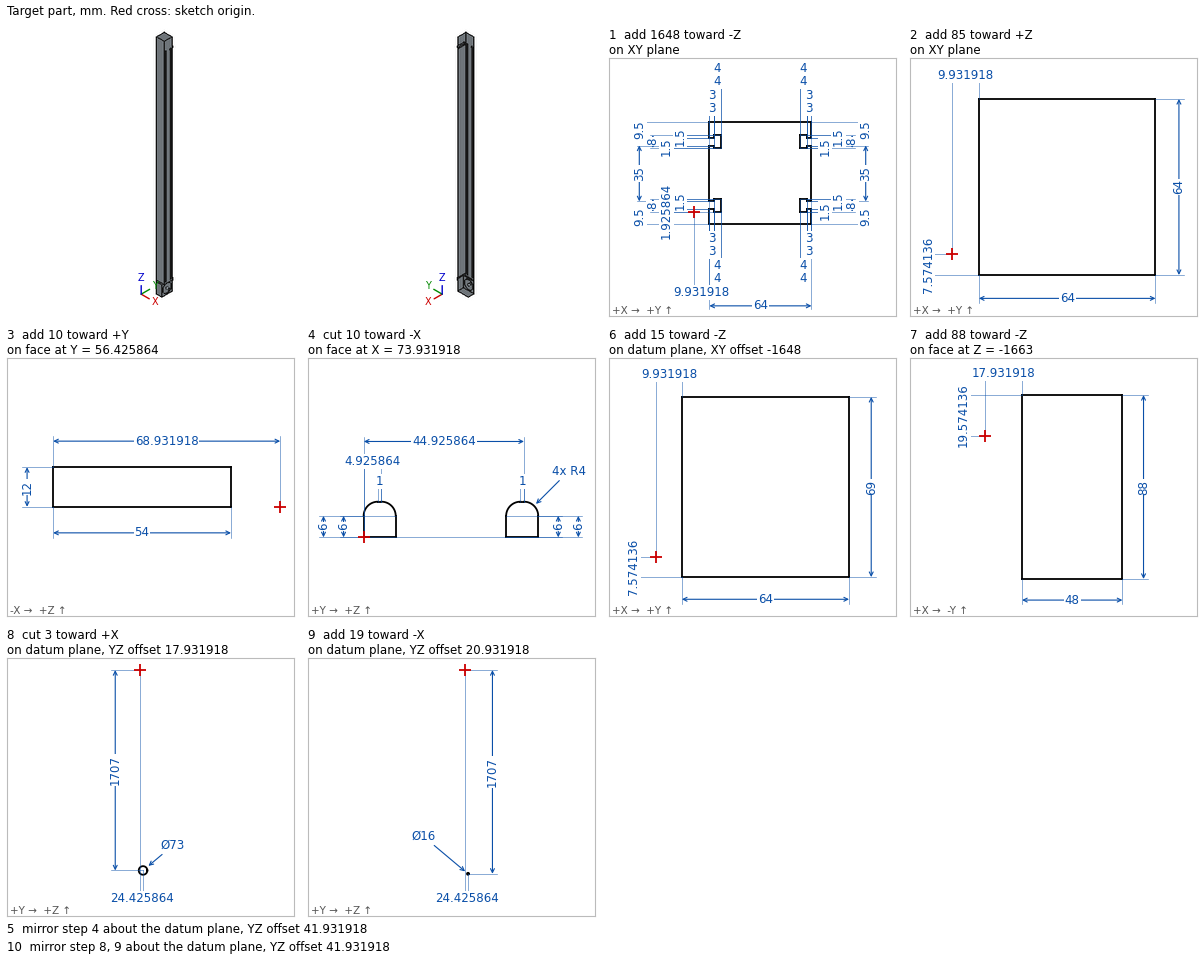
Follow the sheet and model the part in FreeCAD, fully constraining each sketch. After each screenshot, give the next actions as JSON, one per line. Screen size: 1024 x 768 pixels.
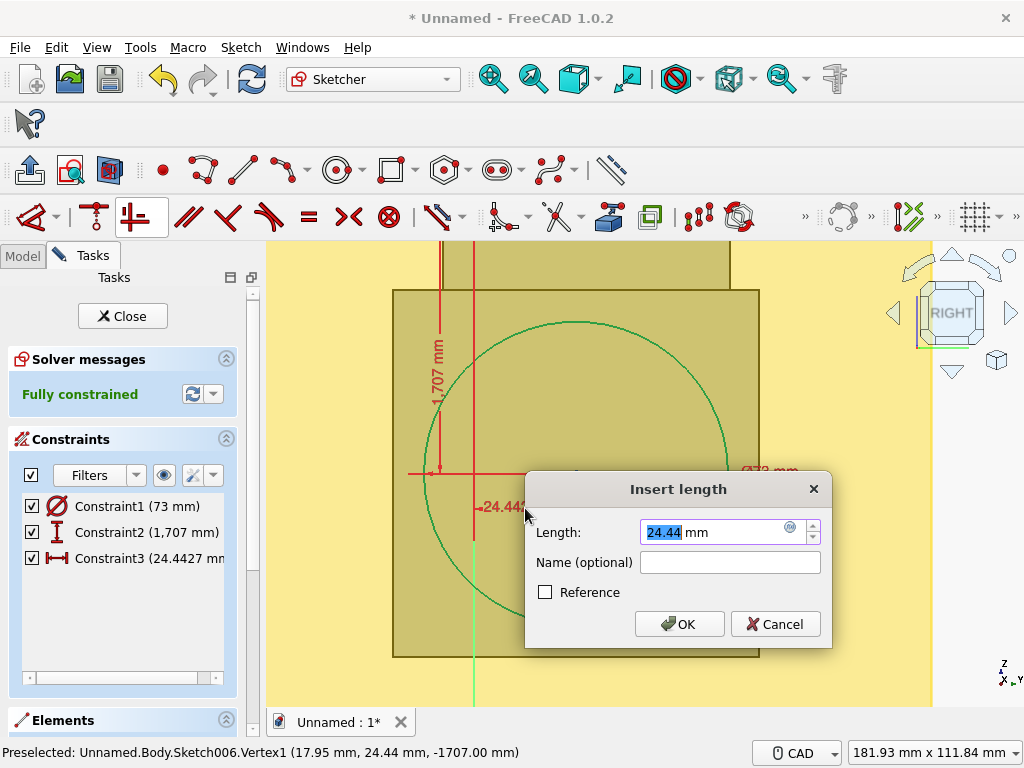
{"action": "type", "text": "24.425864"}
{"action": "key", "text": "Return"}
{"action": "key", "text": "Escape"}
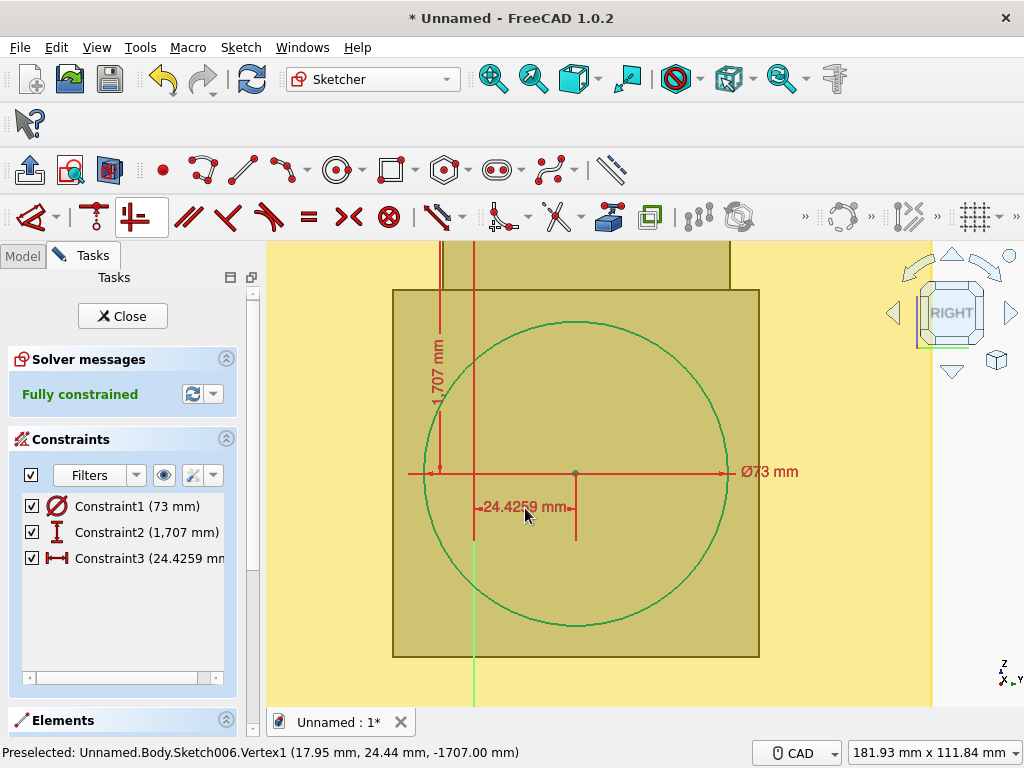
{"action": "left_click", "coordinate": [123, 316]}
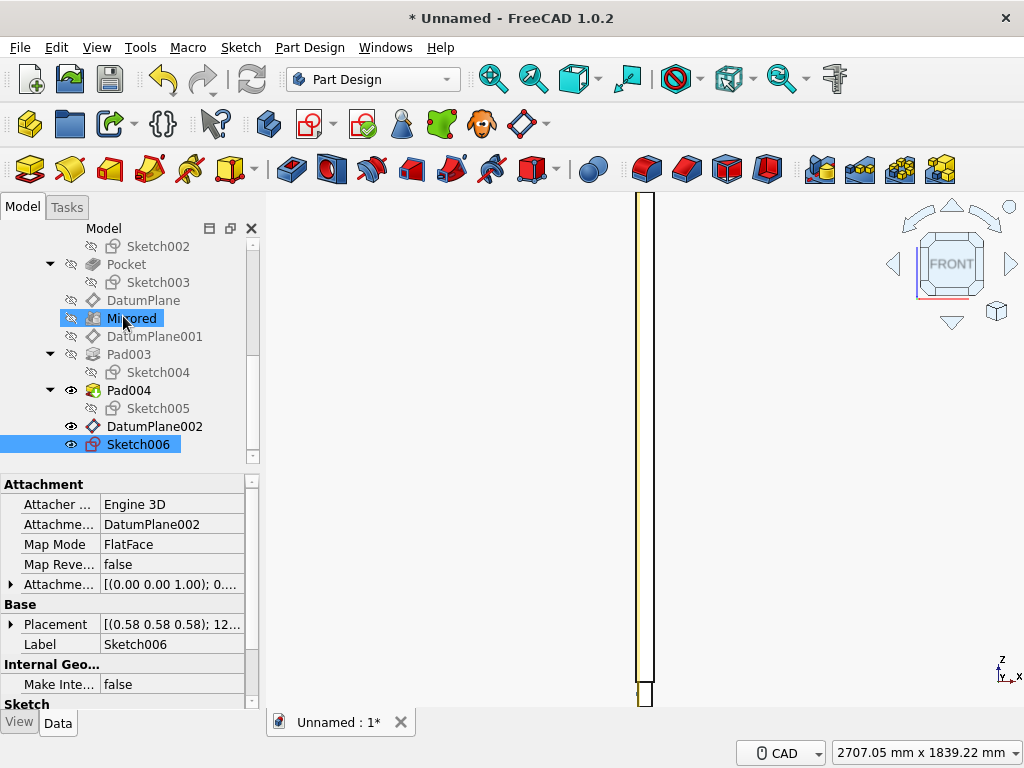
{"action": "left_click", "coordinate": [292, 170]}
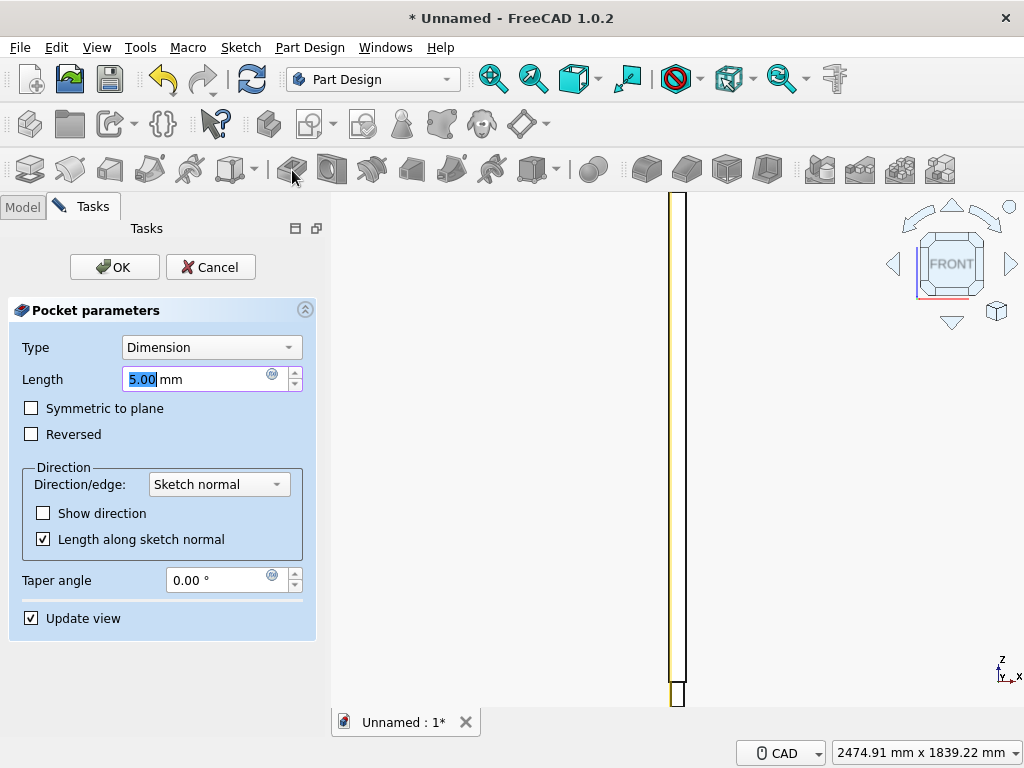
{"action": "type", "text": "3"}
{"action": "key", "text": "Tab"}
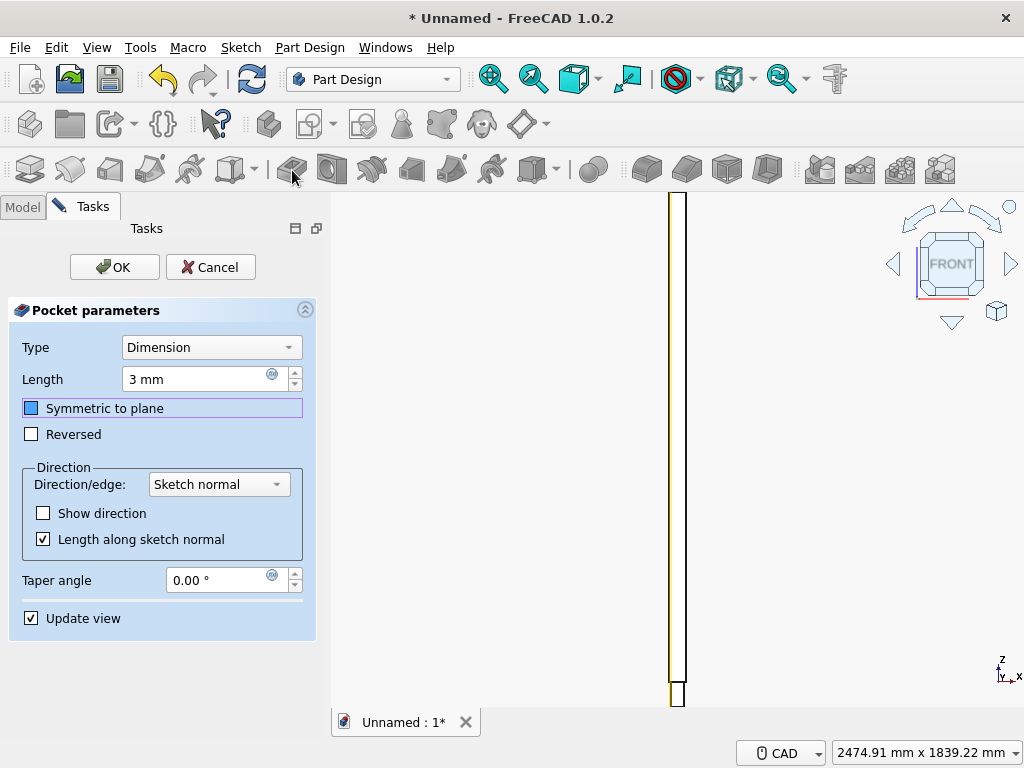
{"action": "left_click", "coordinate": [30, 434]}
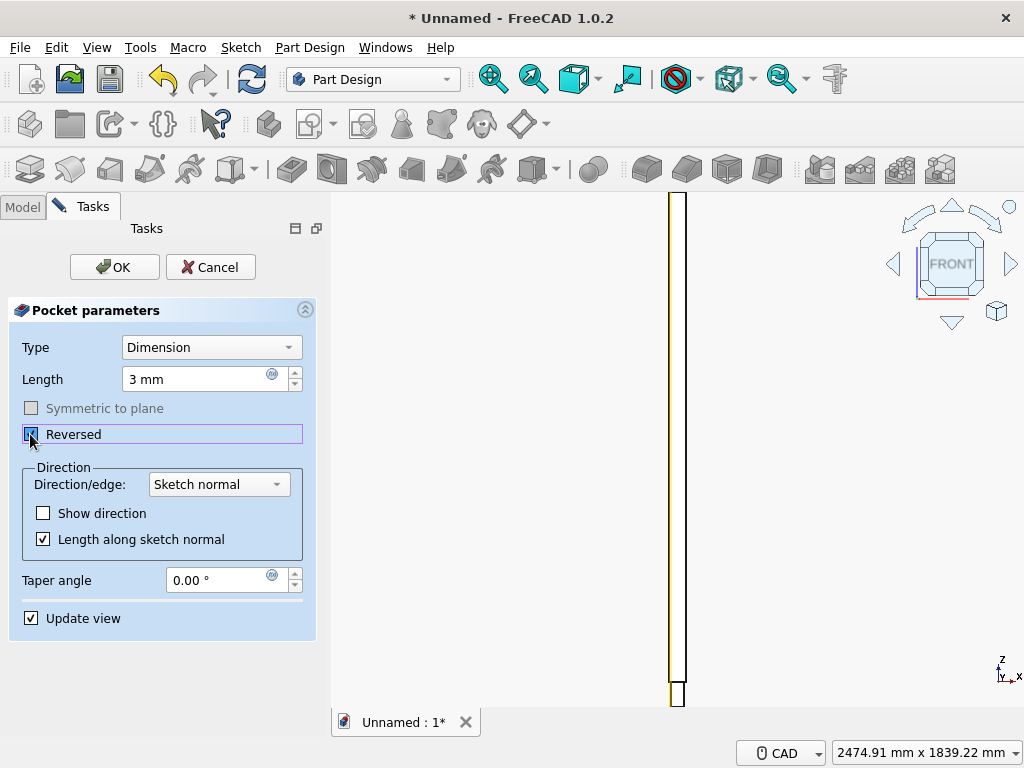
{"action": "left_click", "coordinate": [115, 267]}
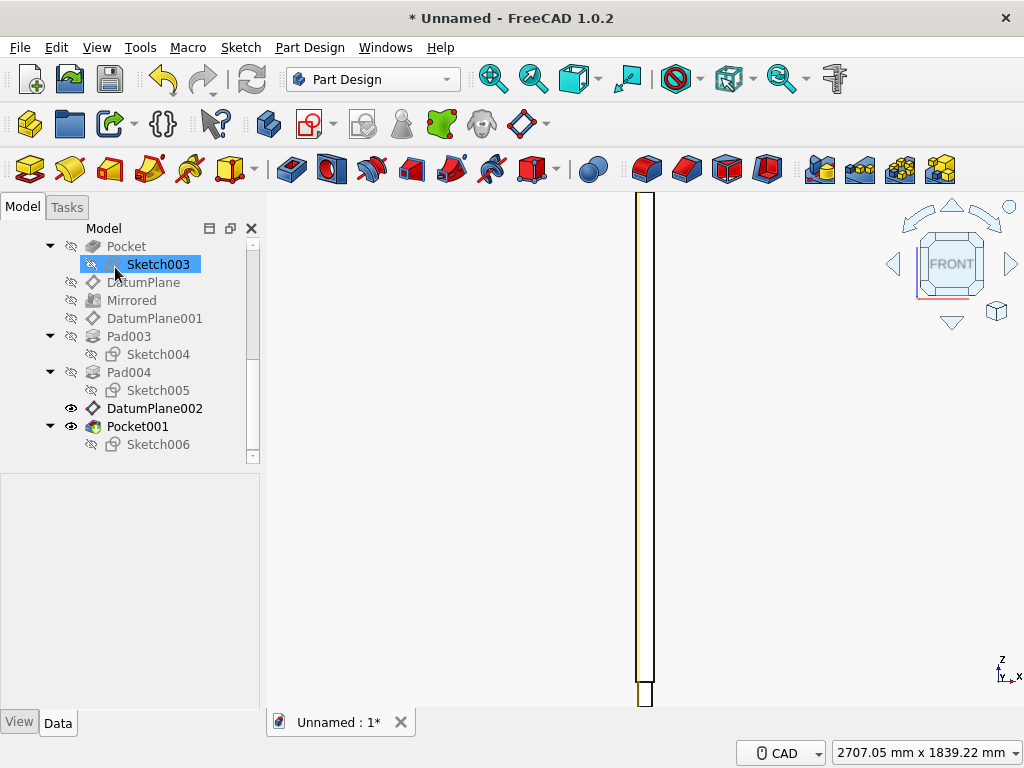
{"action": "left_click", "coordinate": [116, 408]}
{"action": "key", "text": "space"}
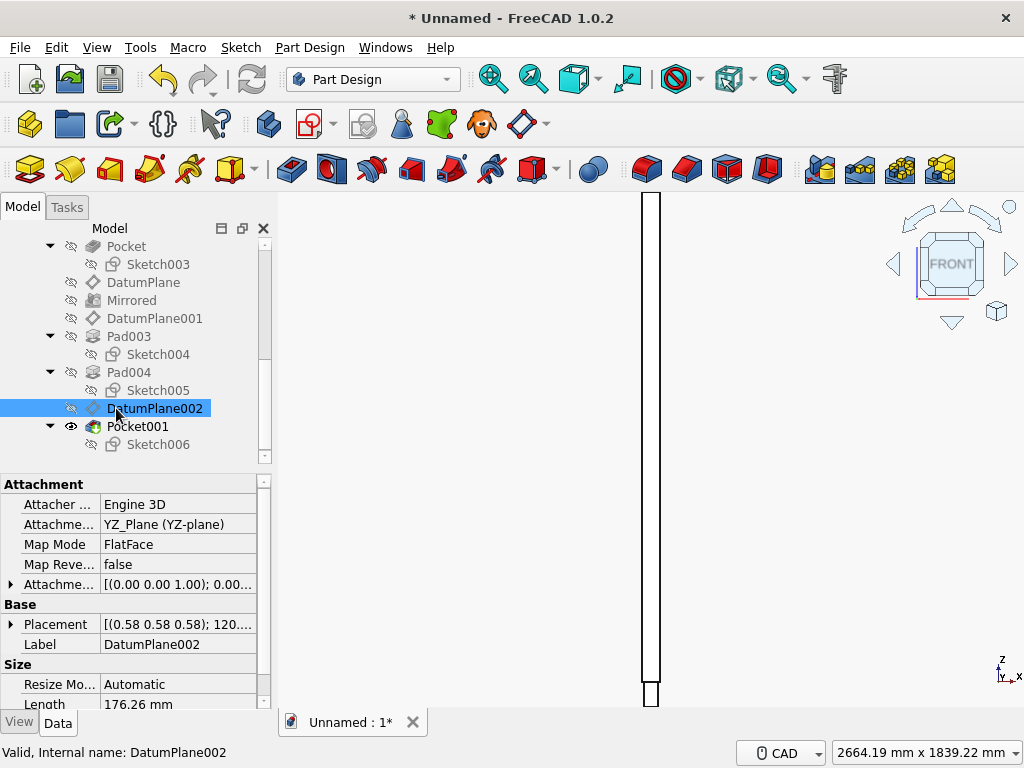
{"action": "left_click", "coordinate": [494, 80]}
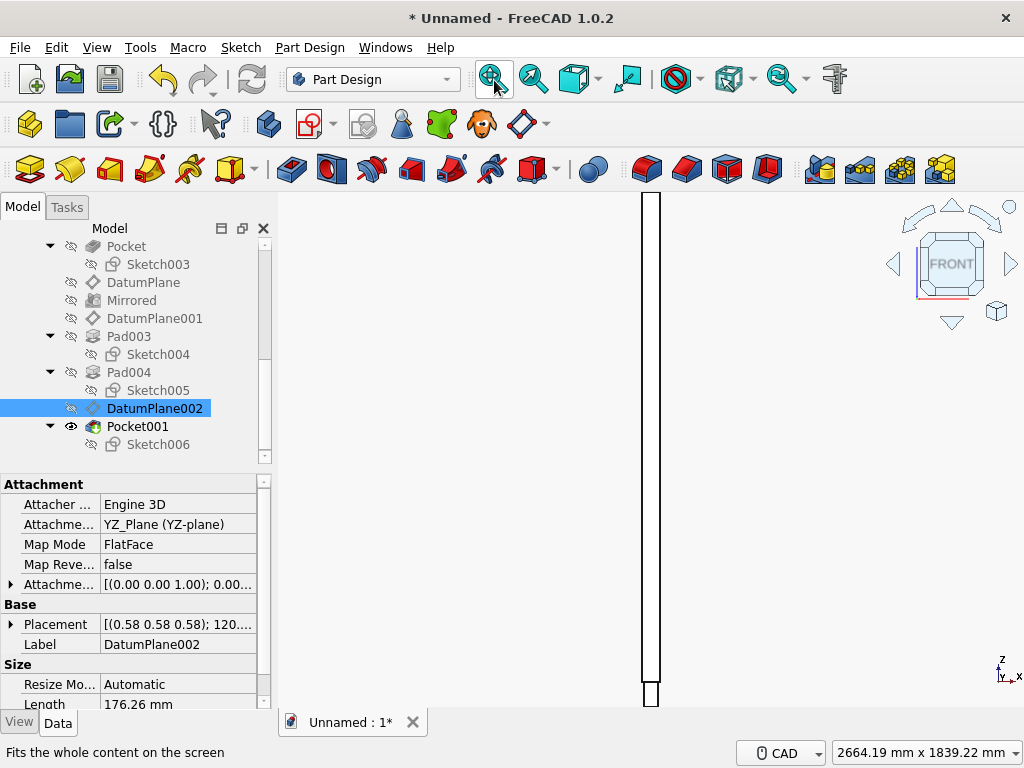
{"action": "key", "text": "6"}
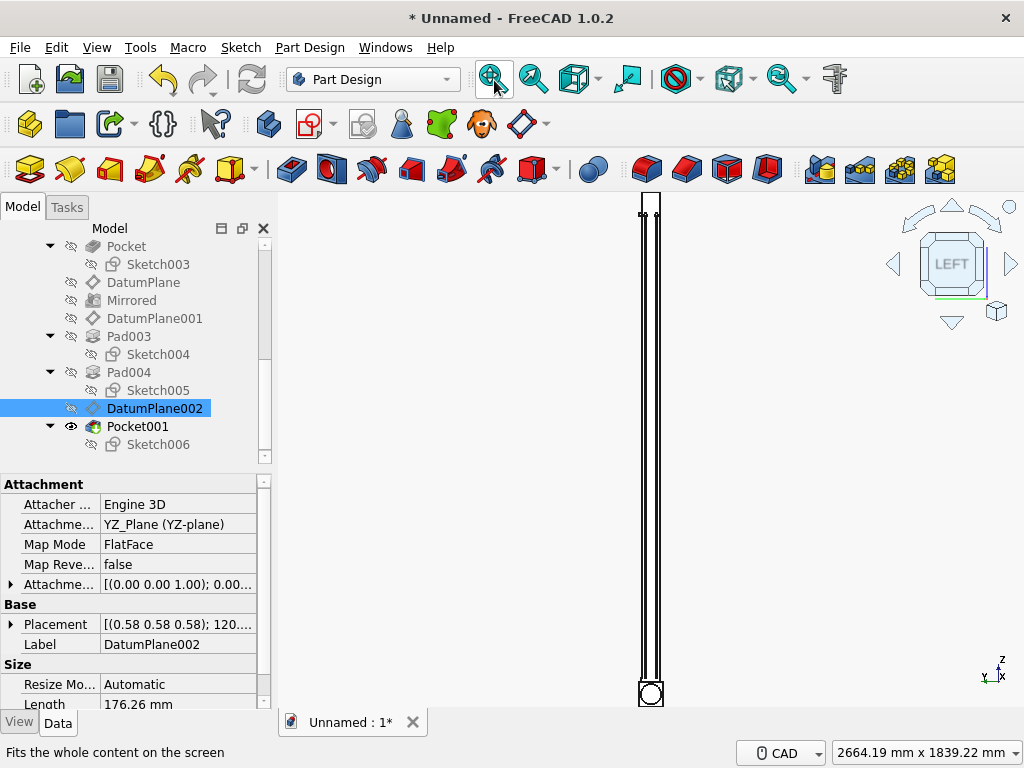
{"action": "left_click", "coordinate": [494, 80]}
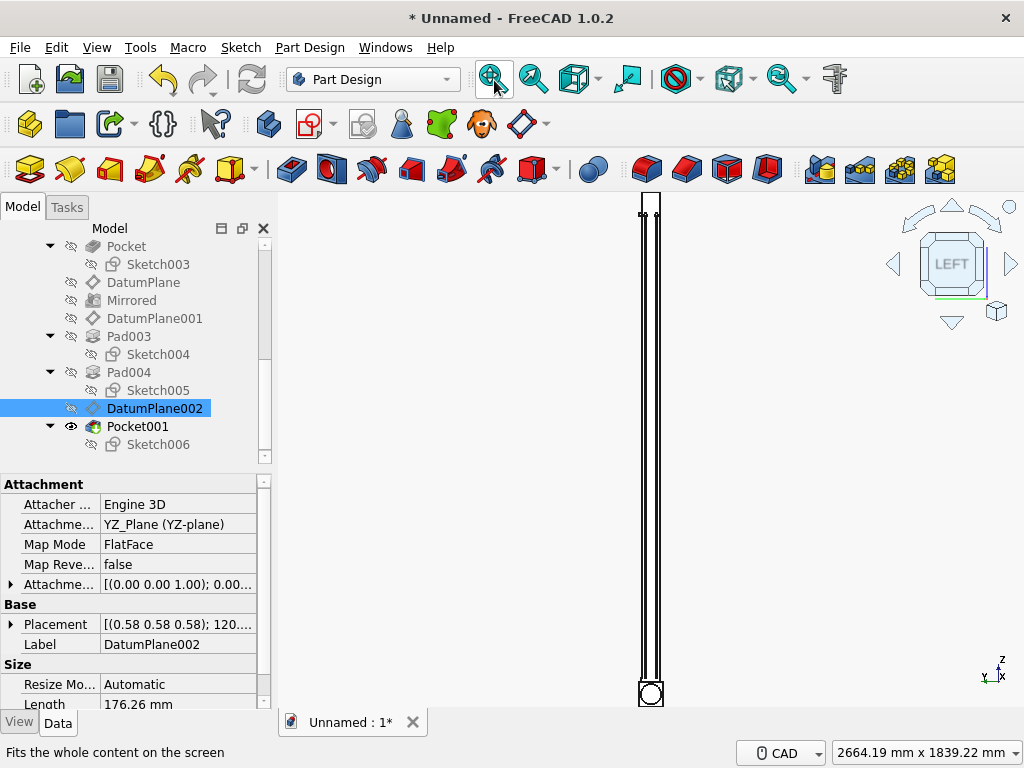
{"action": "key", "text": "2"}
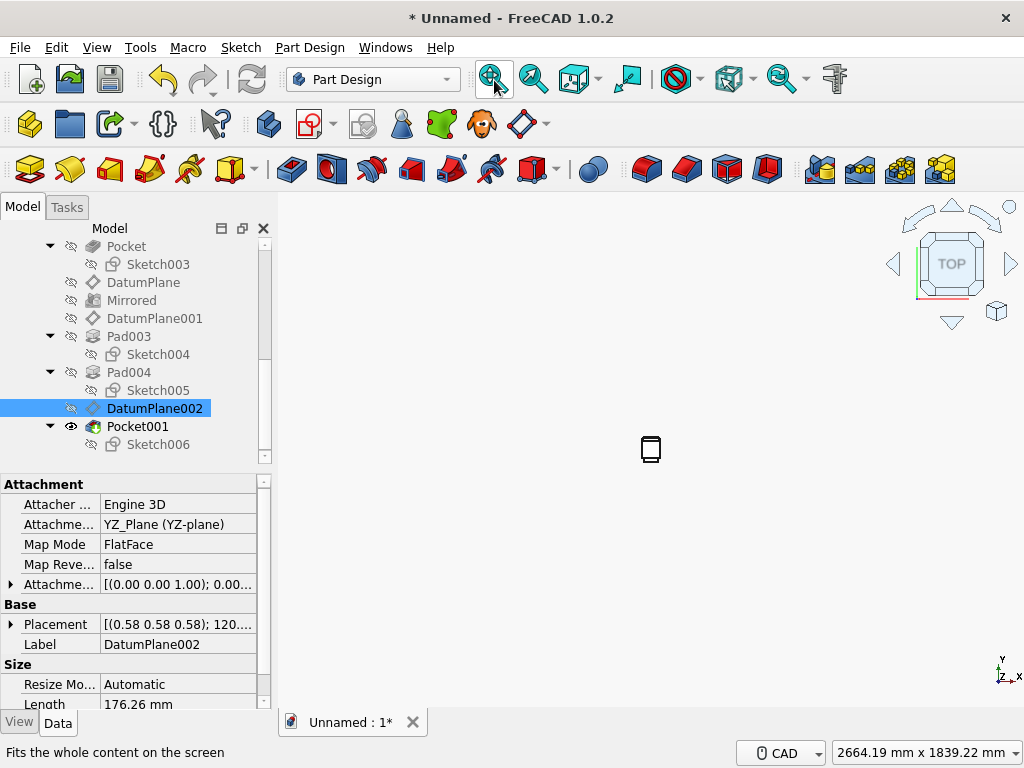
{"action": "left_click", "coordinate": [494, 80]}